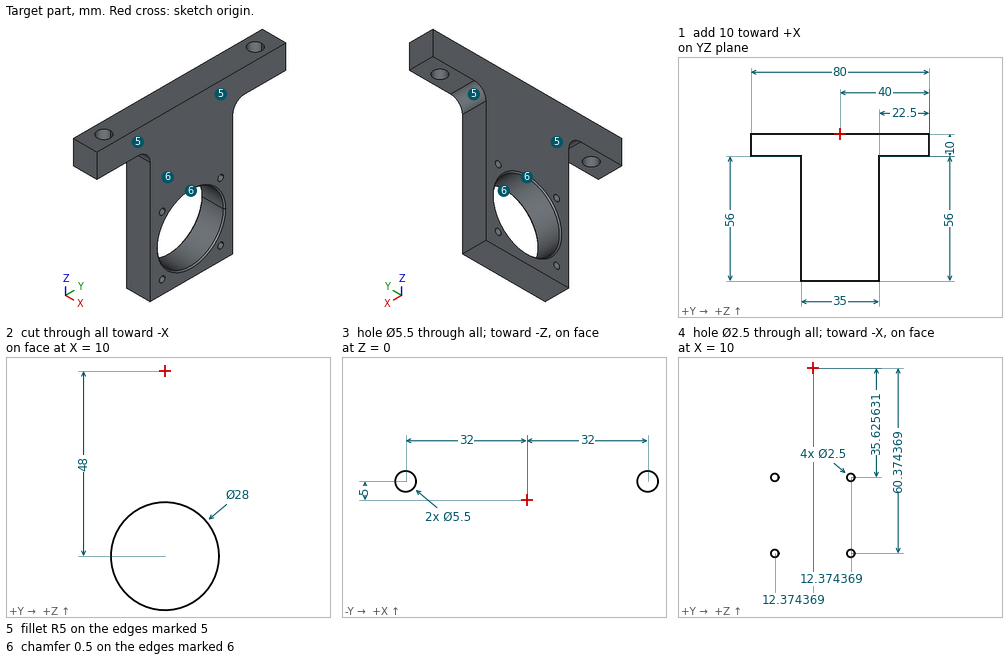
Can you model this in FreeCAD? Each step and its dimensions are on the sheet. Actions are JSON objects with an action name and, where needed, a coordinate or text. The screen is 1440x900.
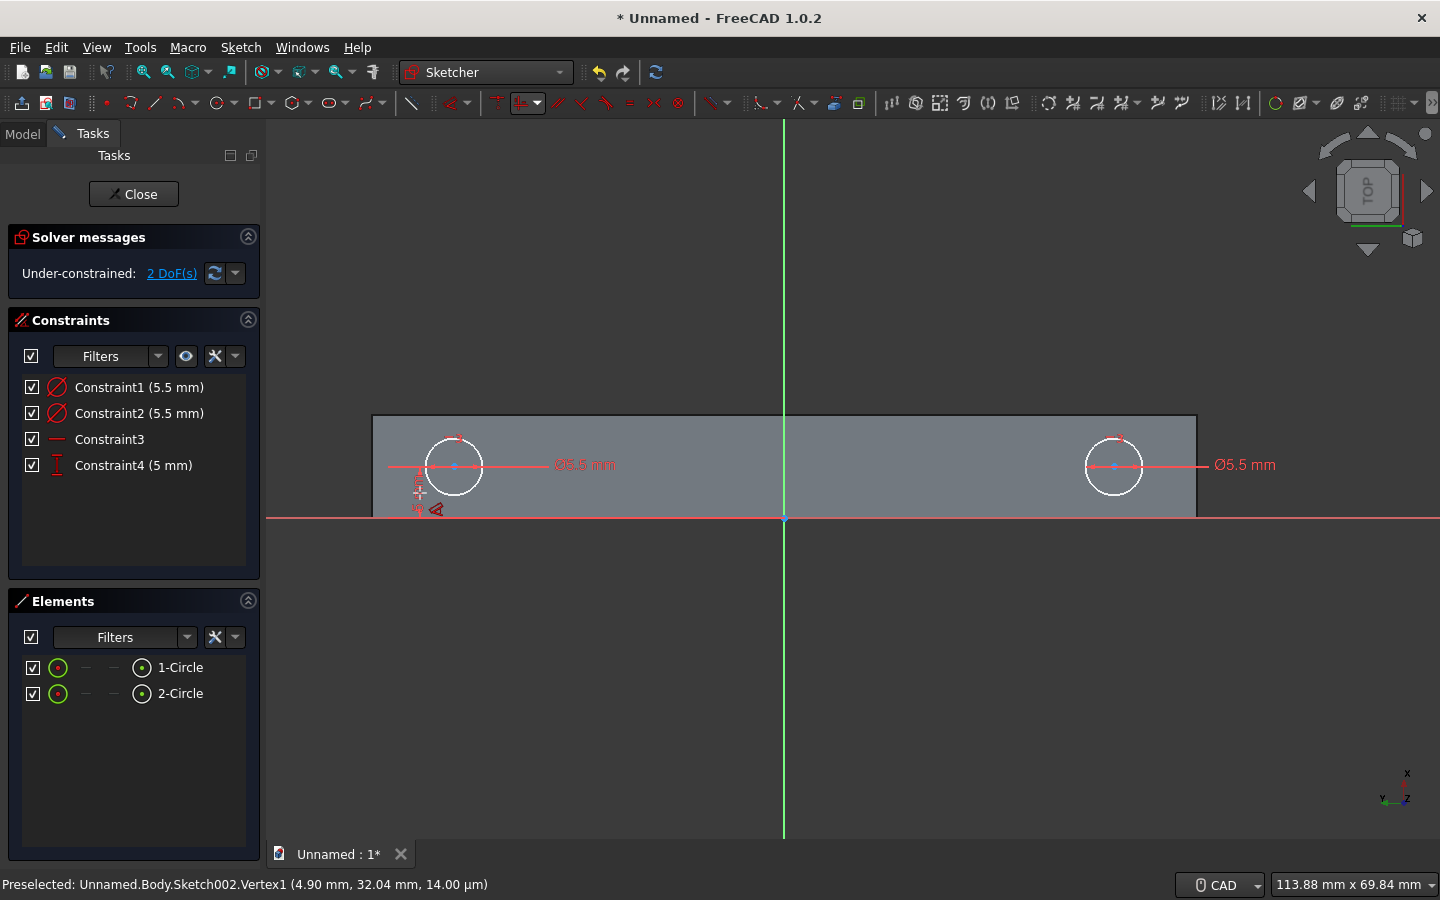
{"action": "left_click", "coordinate": [454, 467]}
{"action": "left_click", "coordinate": [619, 552]}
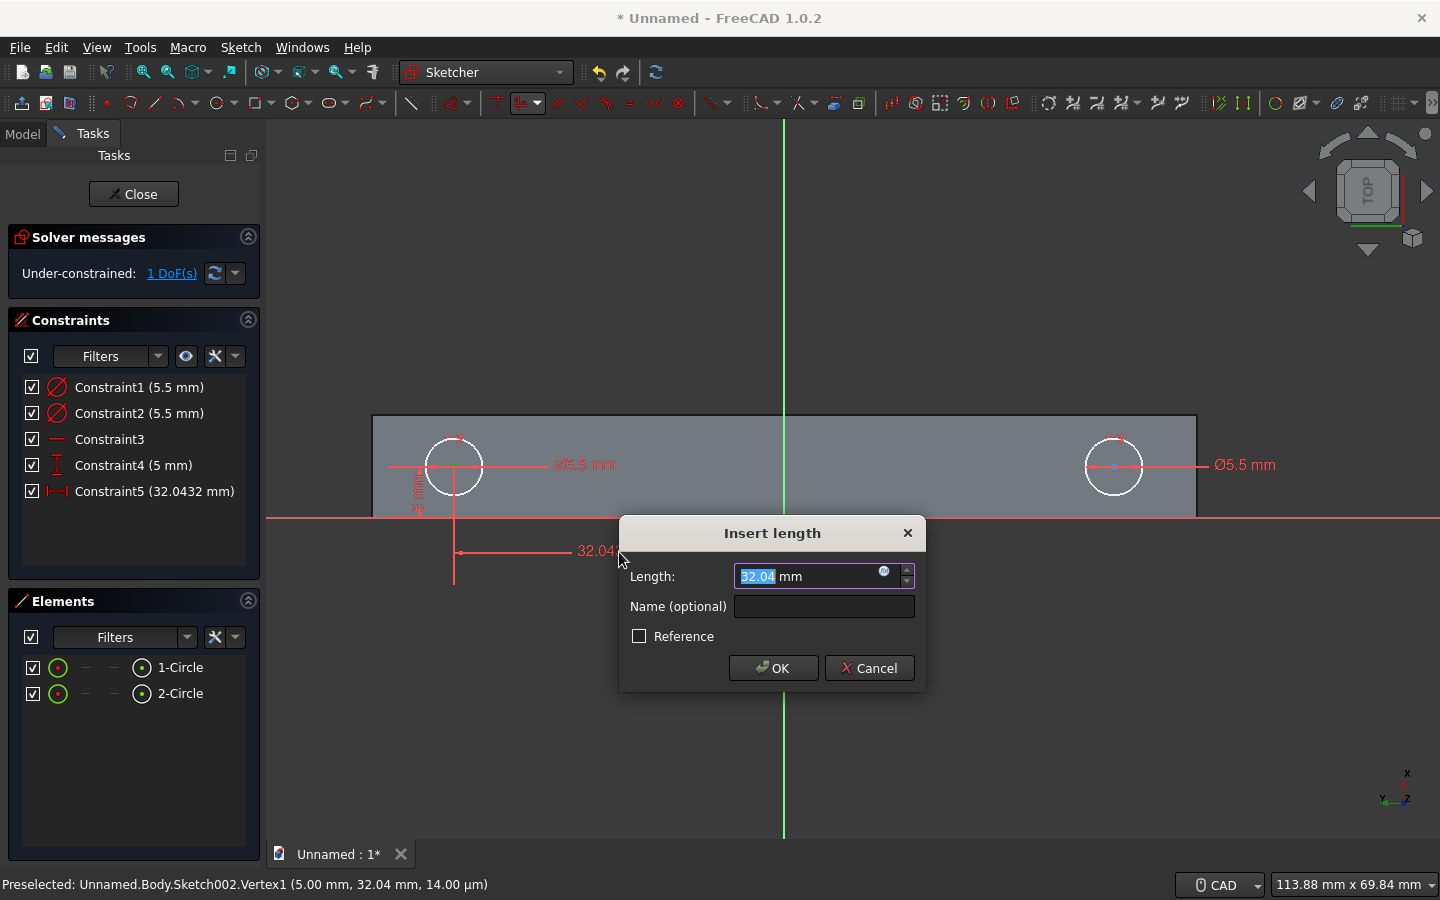
{"action": "type", "text": "32"}
{"action": "key", "text": "Return"}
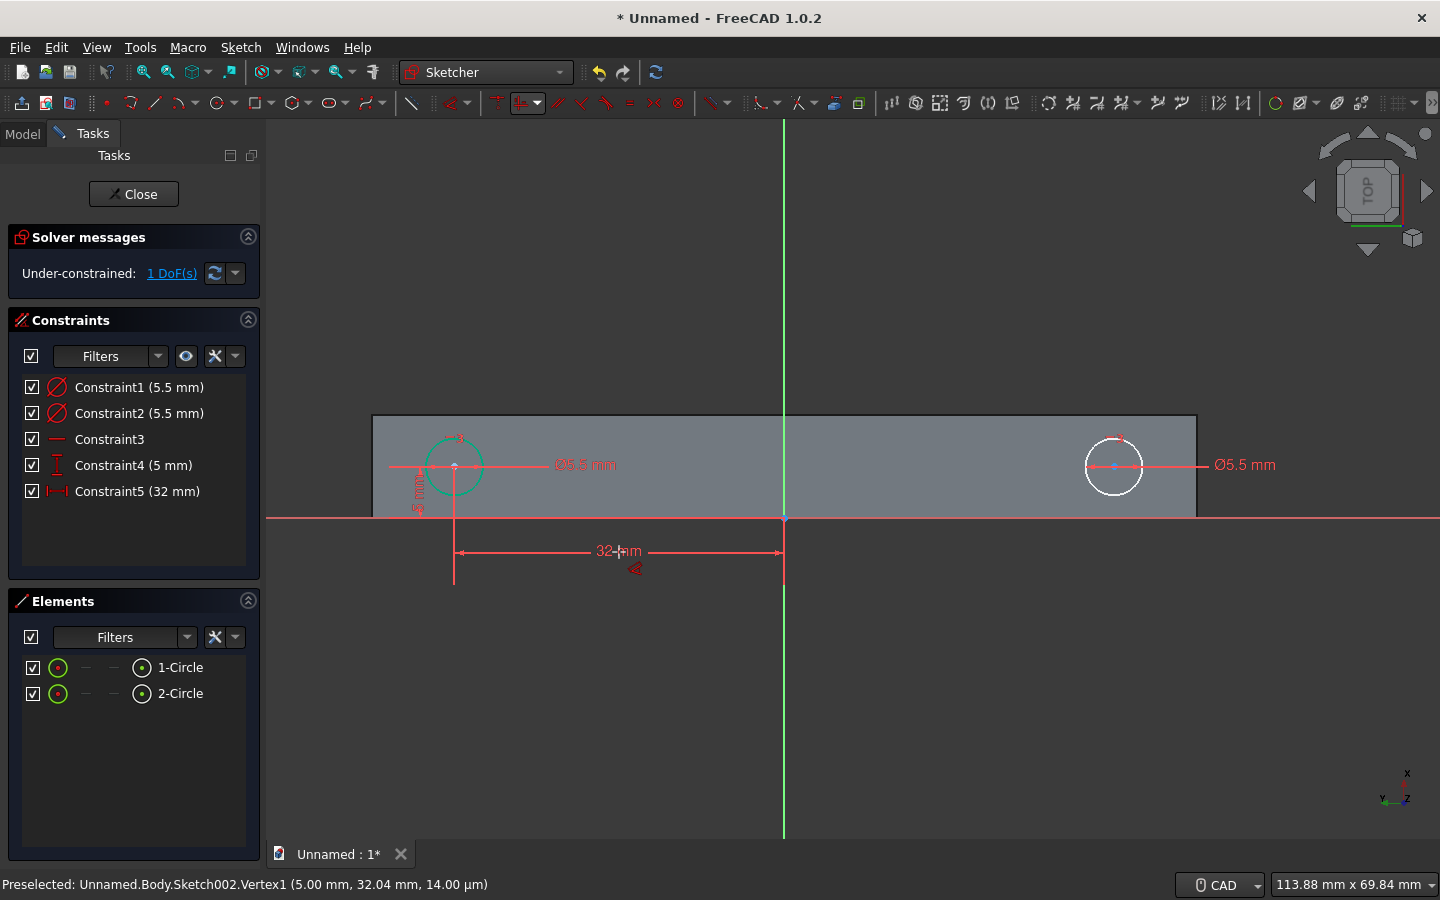
{"action": "left_click", "coordinate": [1114, 467]}
{"action": "left_click", "coordinate": [949, 552]}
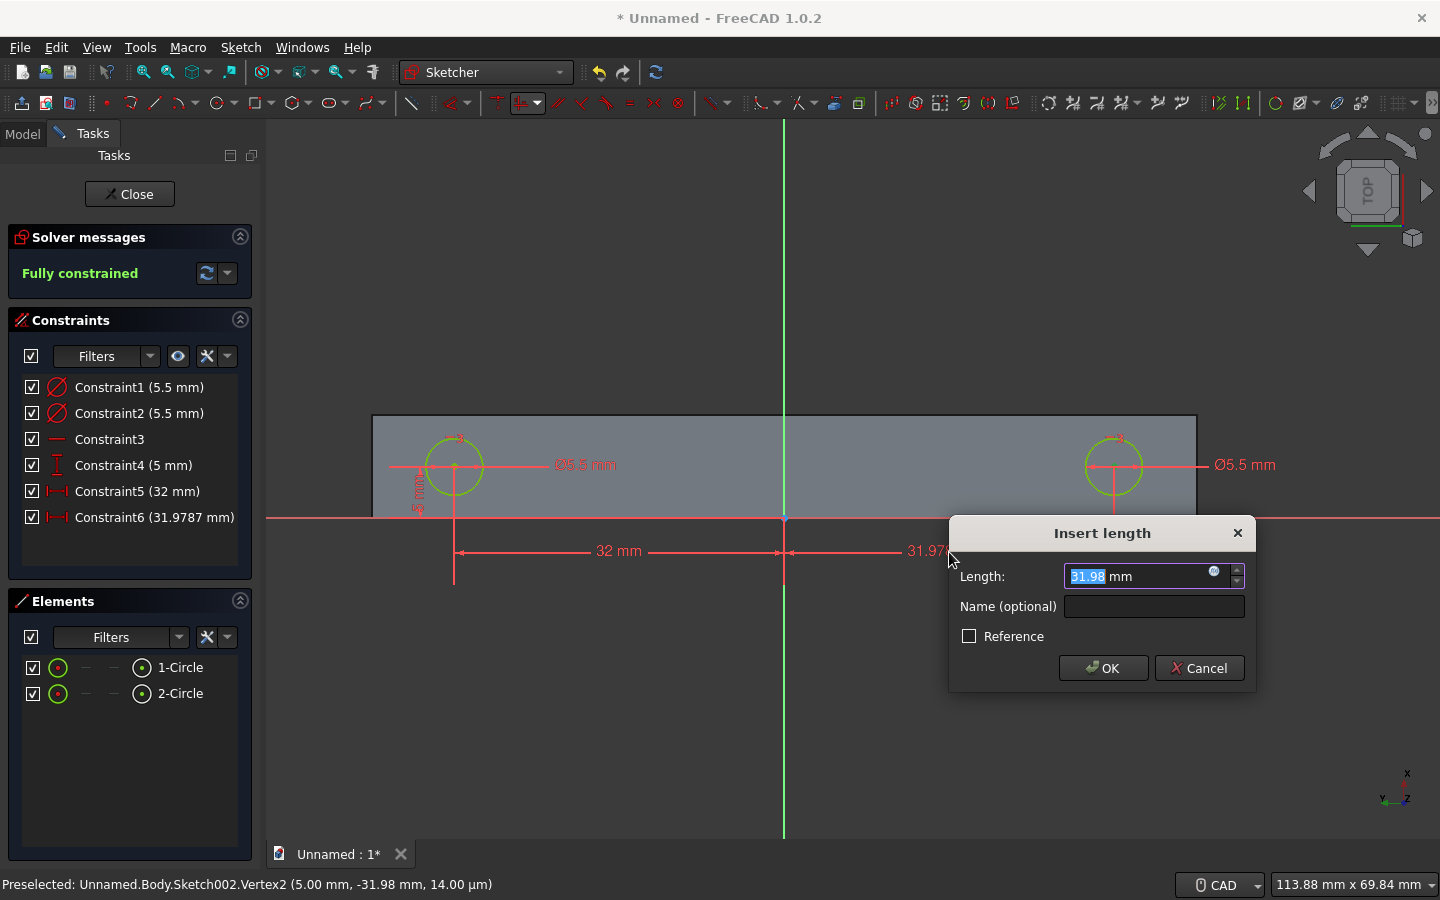
{"action": "type", "text": "32"}
{"action": "key", "text": "Return"}
{"action": "key", "text": "Escape"}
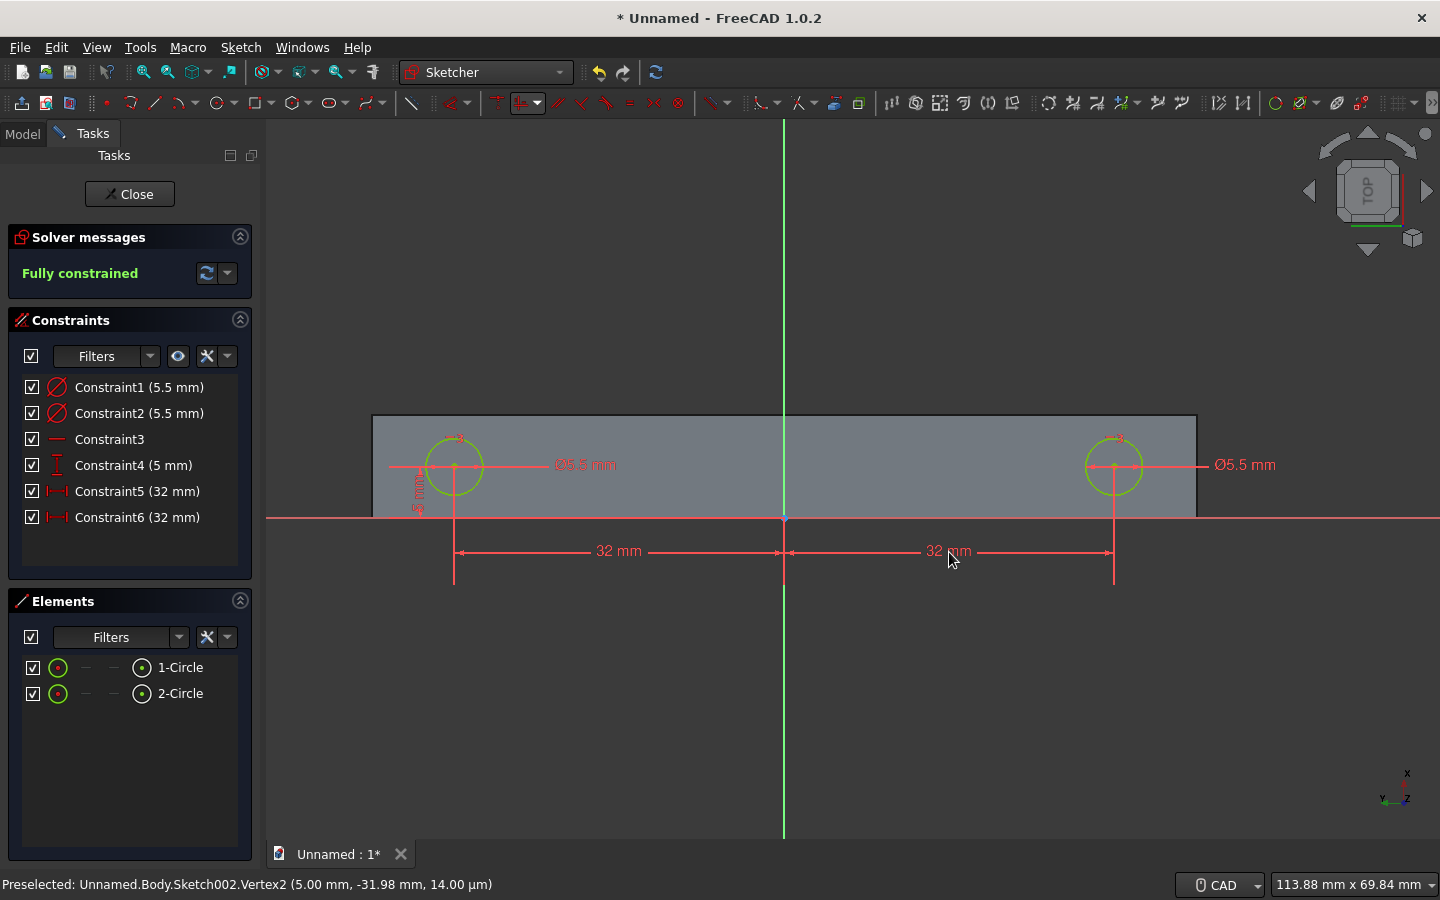
{"action": "left_click", "coordinate": [130, 194]}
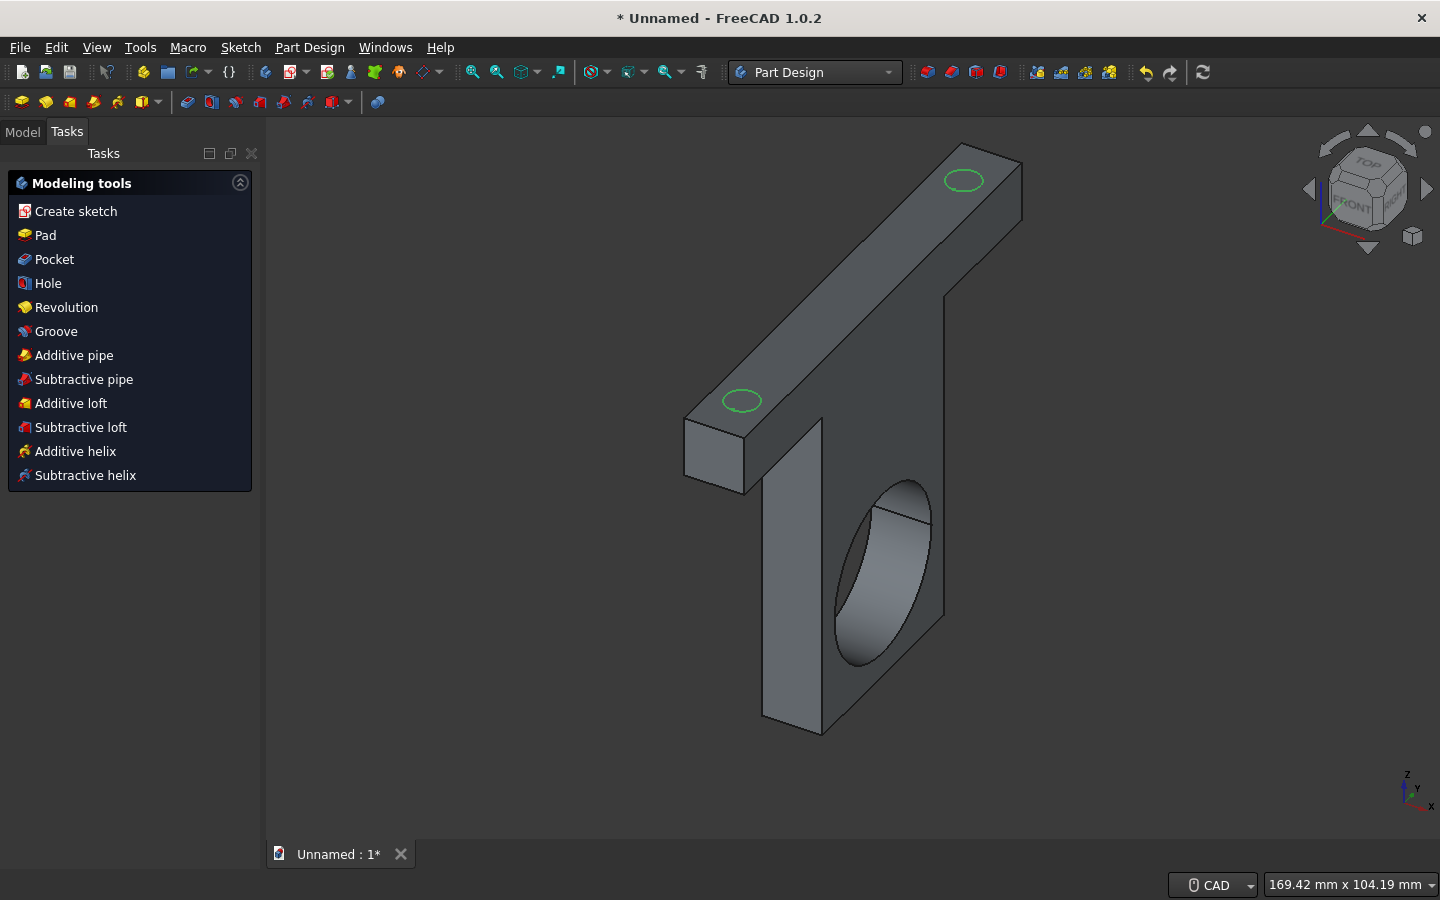
{"action": "left_click", "coordinate": [212, 102]}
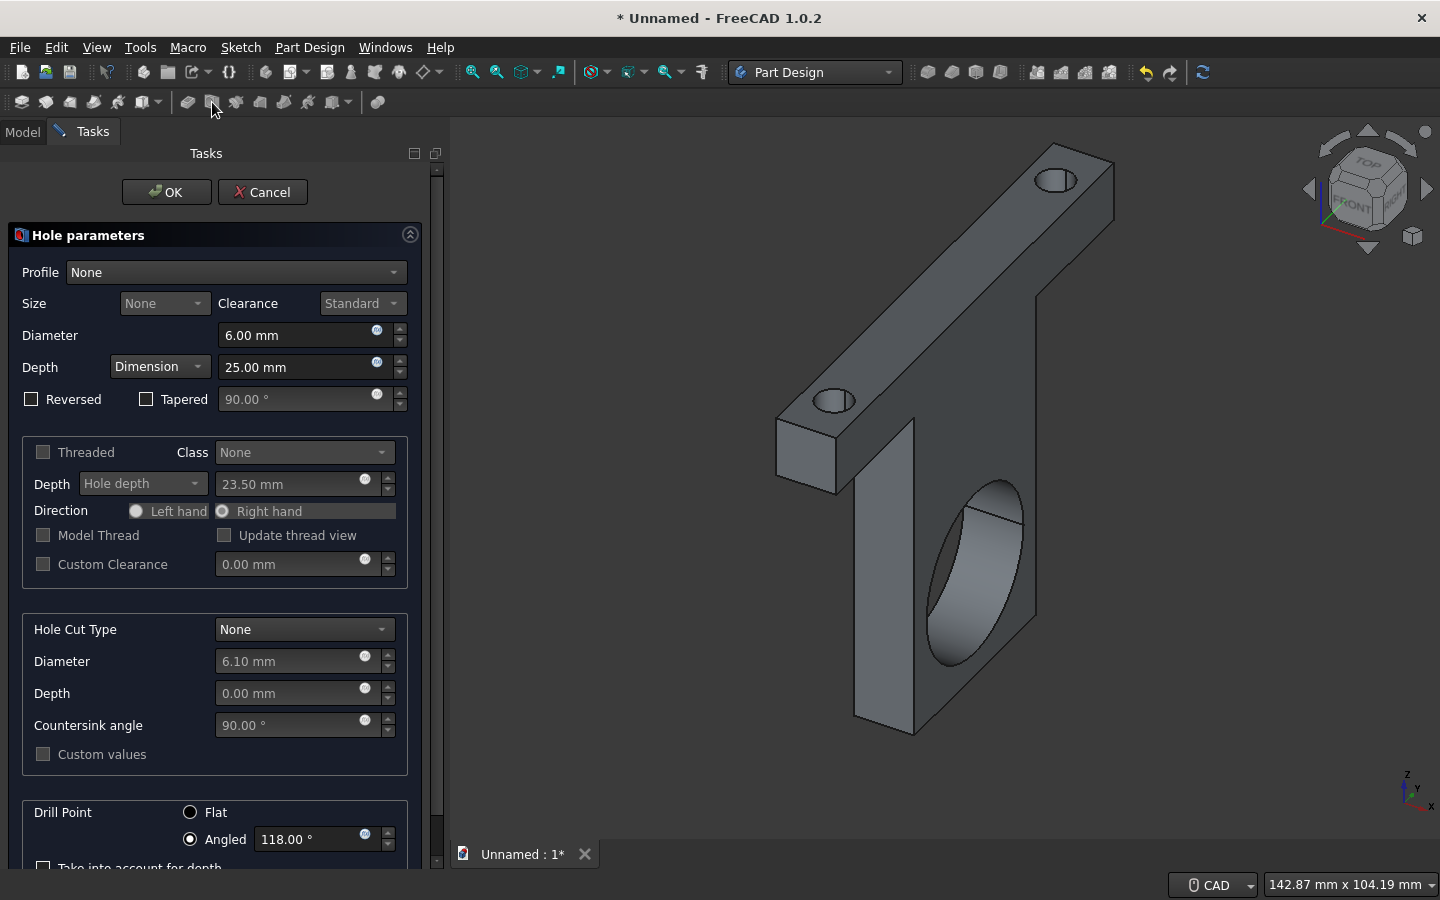
{"action": "triple_click", "coordinate": [305, 335]}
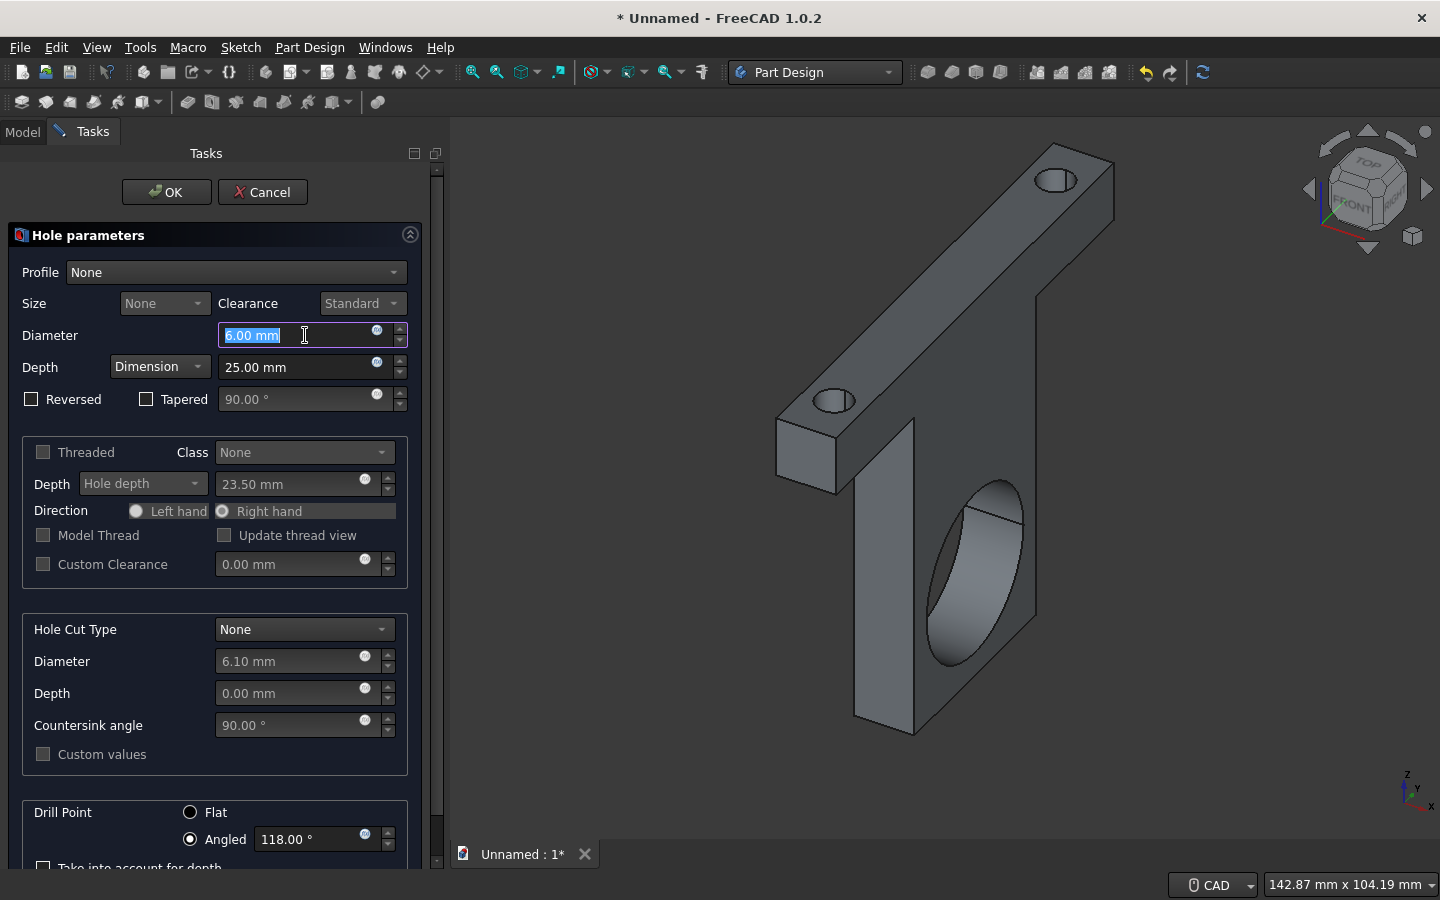
{"action": "type", "text": "5.5"}
{"action": "key", "text": "Tab"}